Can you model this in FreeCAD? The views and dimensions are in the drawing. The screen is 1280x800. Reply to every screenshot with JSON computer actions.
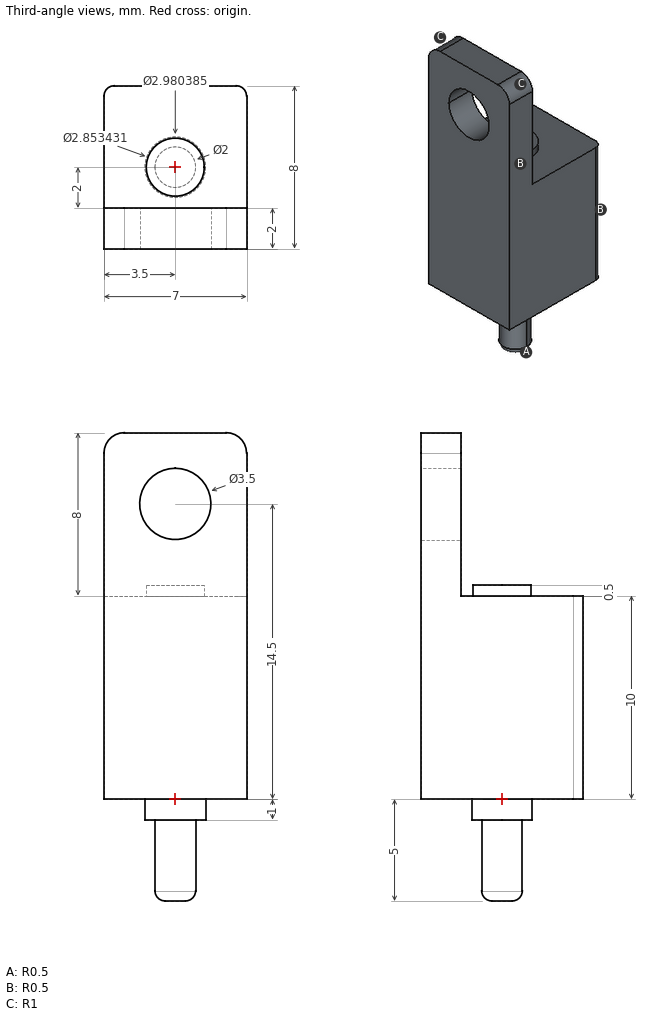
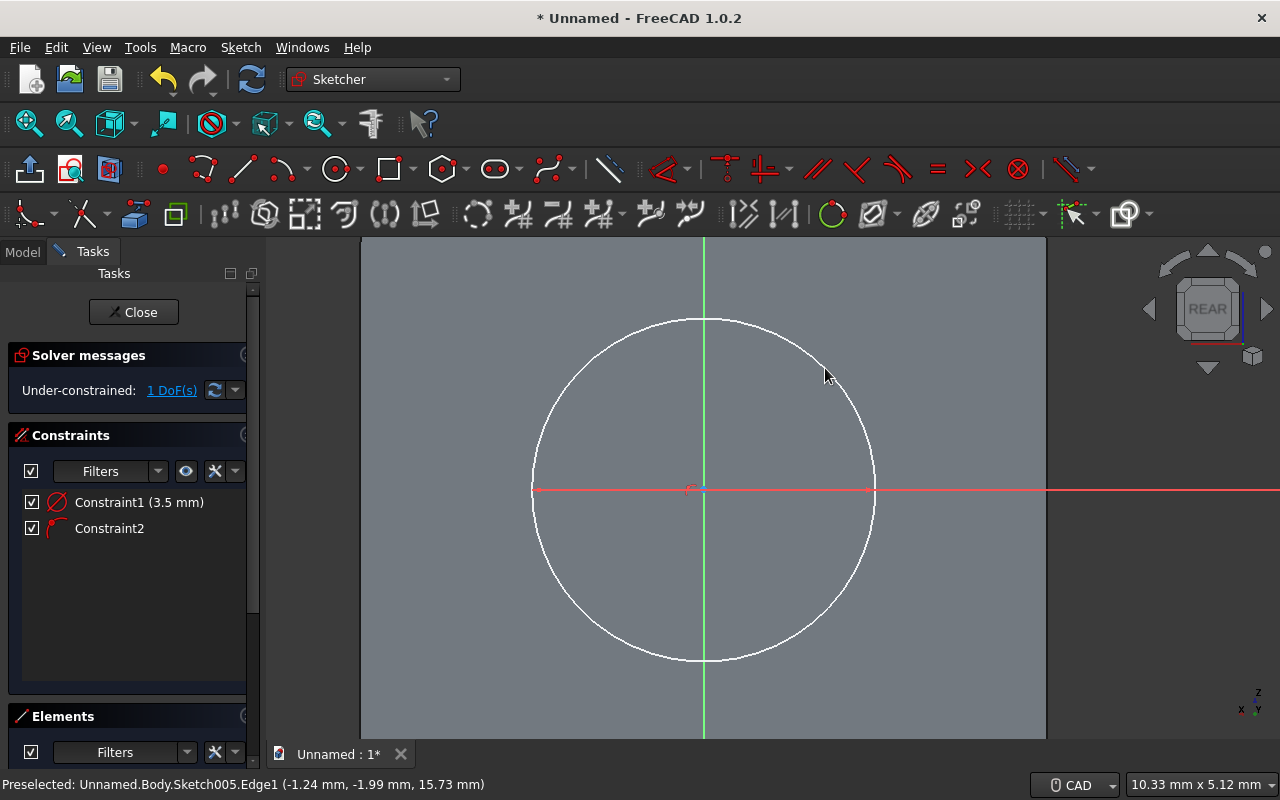
{"action": "key", "text": "d"}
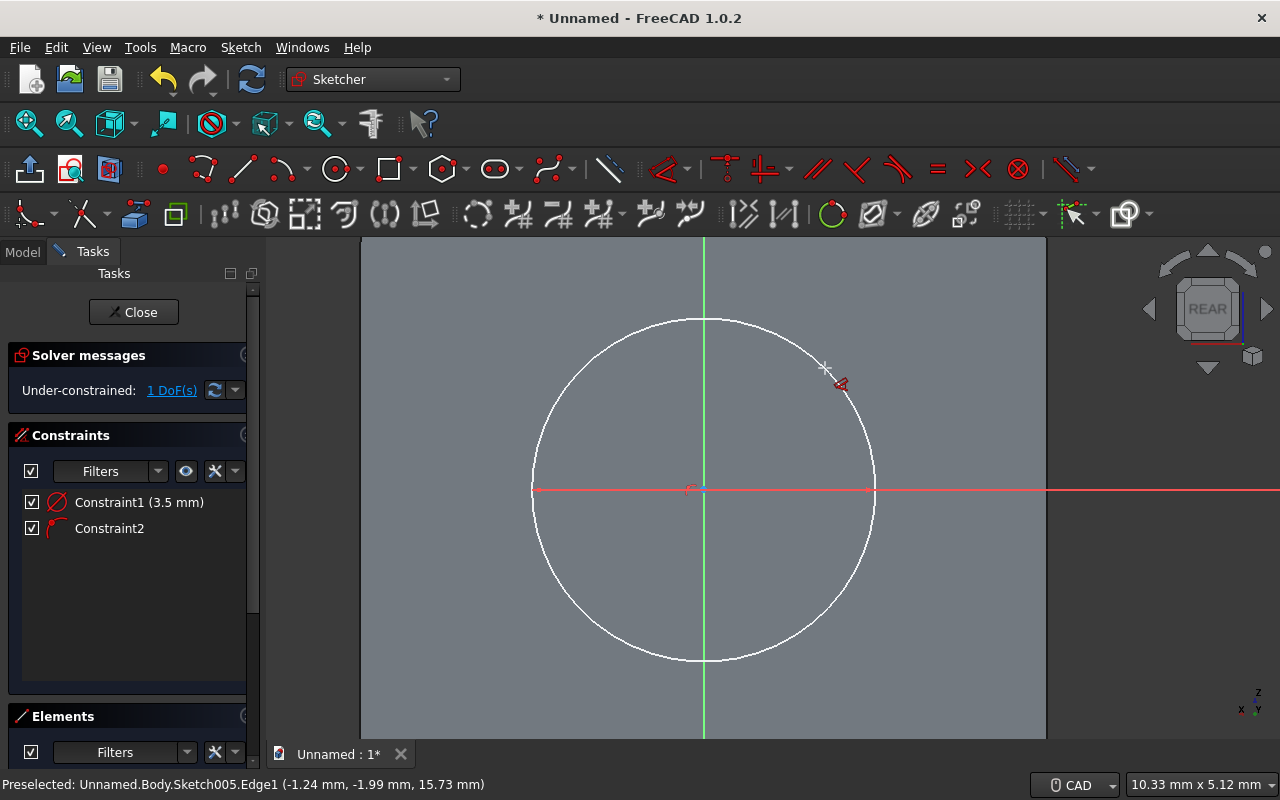
{"action": "left_click", "coordinate": [704, 490]}
{"action": "left_click", "coordinate": [738, 601]}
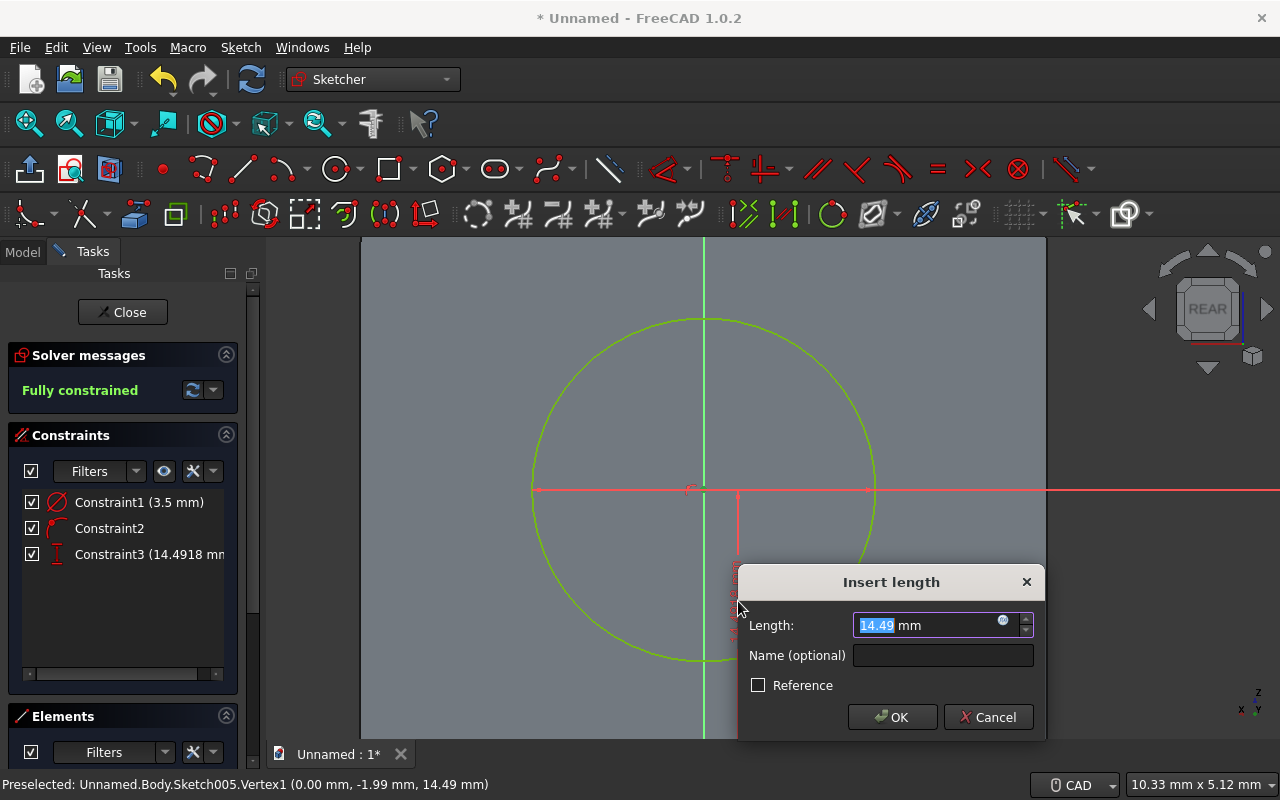
{"action": "type", "text": "14.5"}
{"action": "key", "text": "Return"}
{"action": "key", "text": "Escape"}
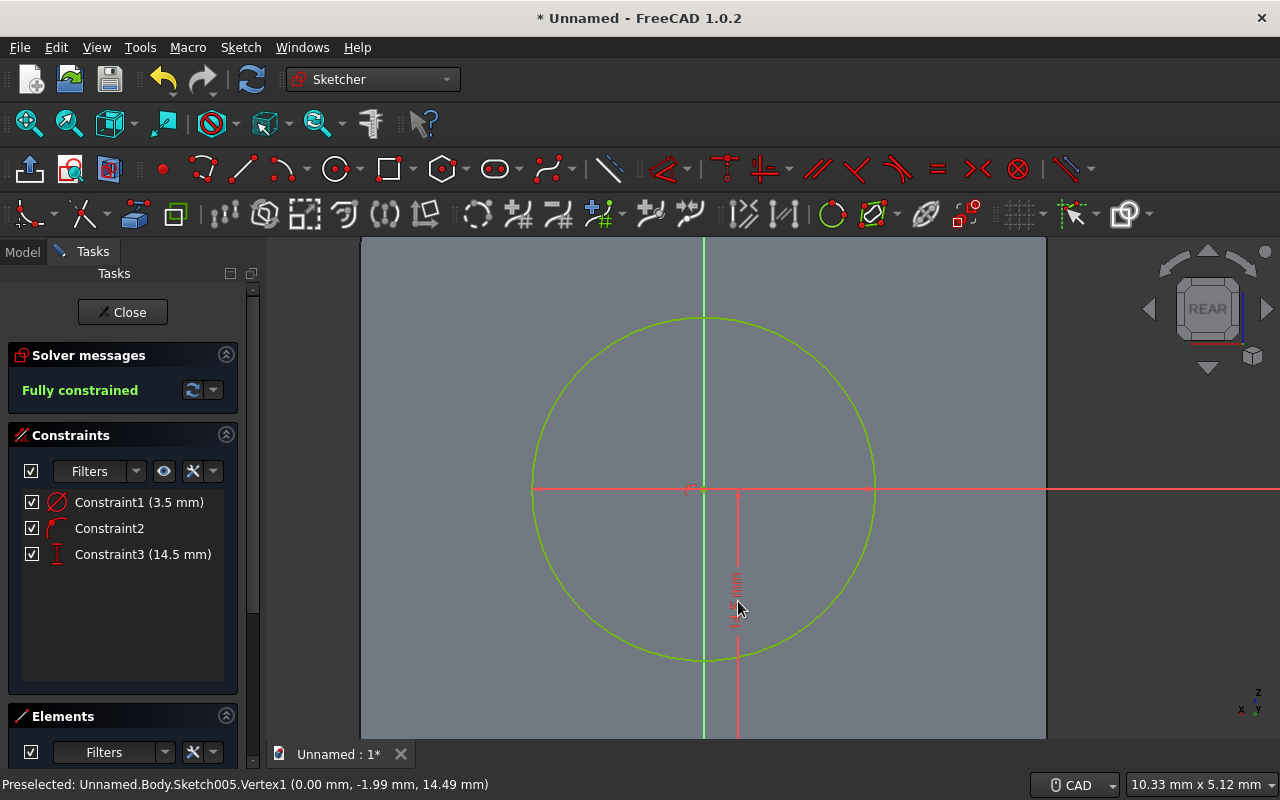
{"action": "left_click", "coordinate": [123, 312]}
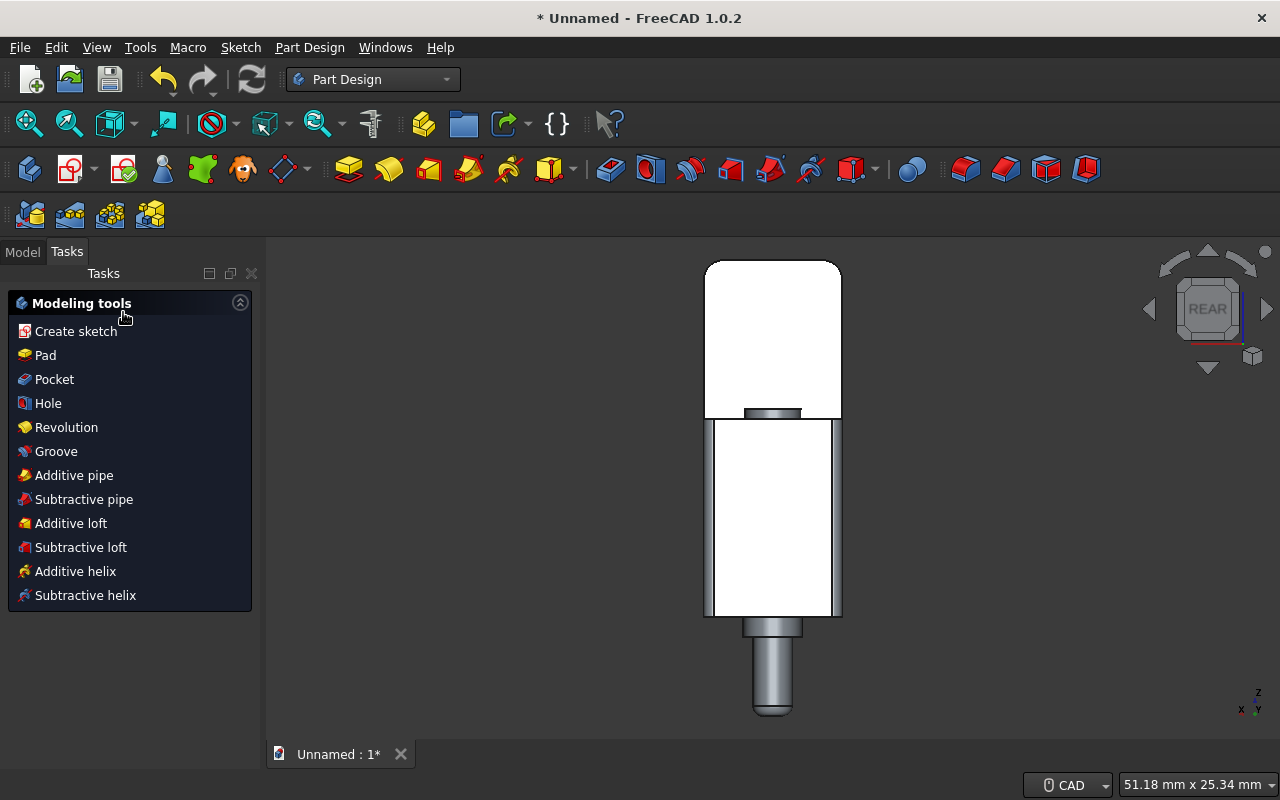
{"action": "left_click", "coordinate": [612, 170]}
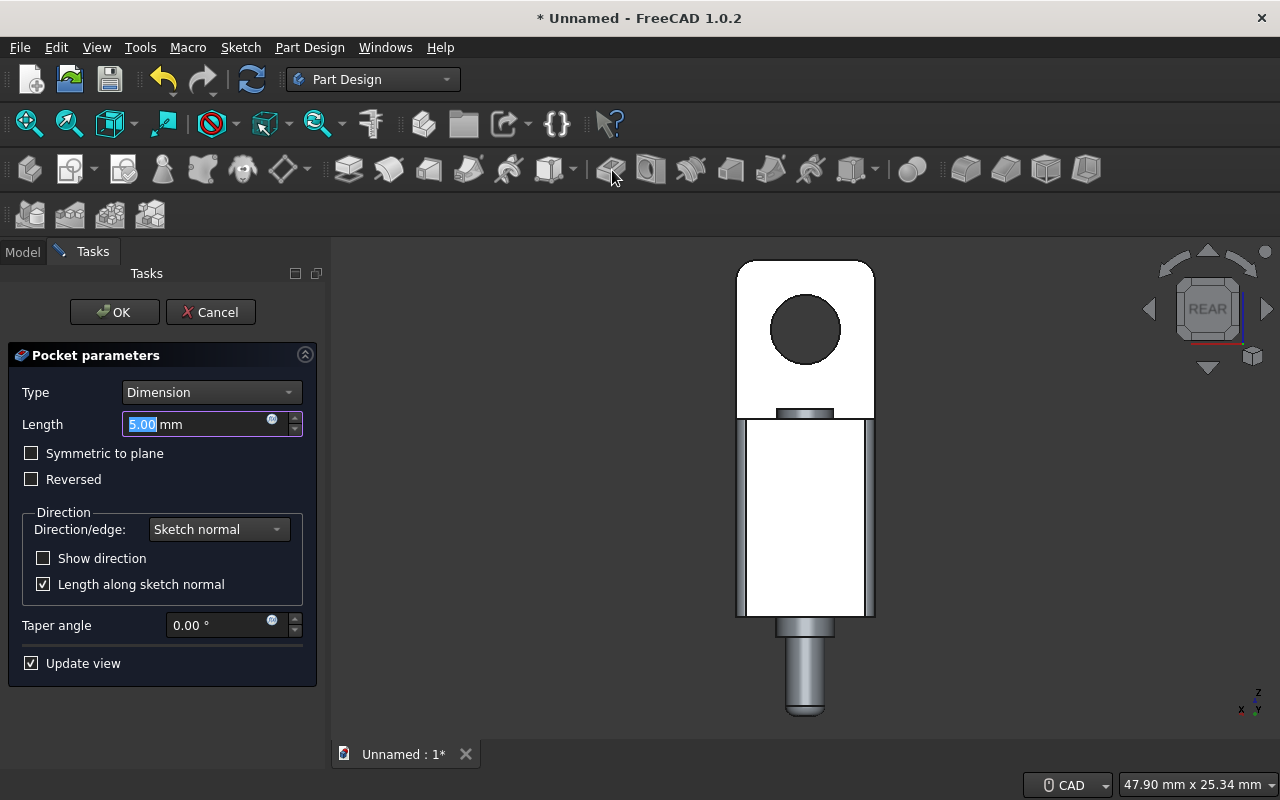
{"action": "left_click", "coordinate": [212, 392]}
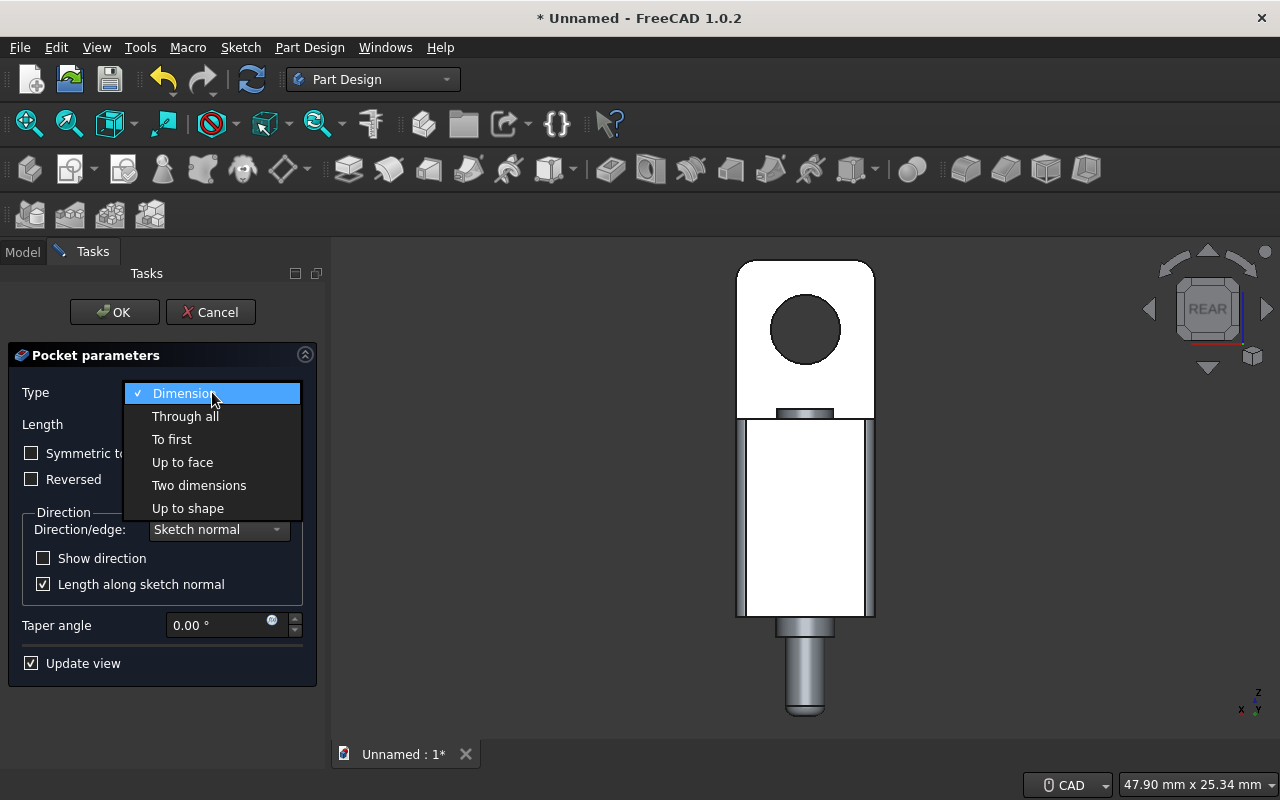
{"action": "left_click", "coordinate": [212, 416]}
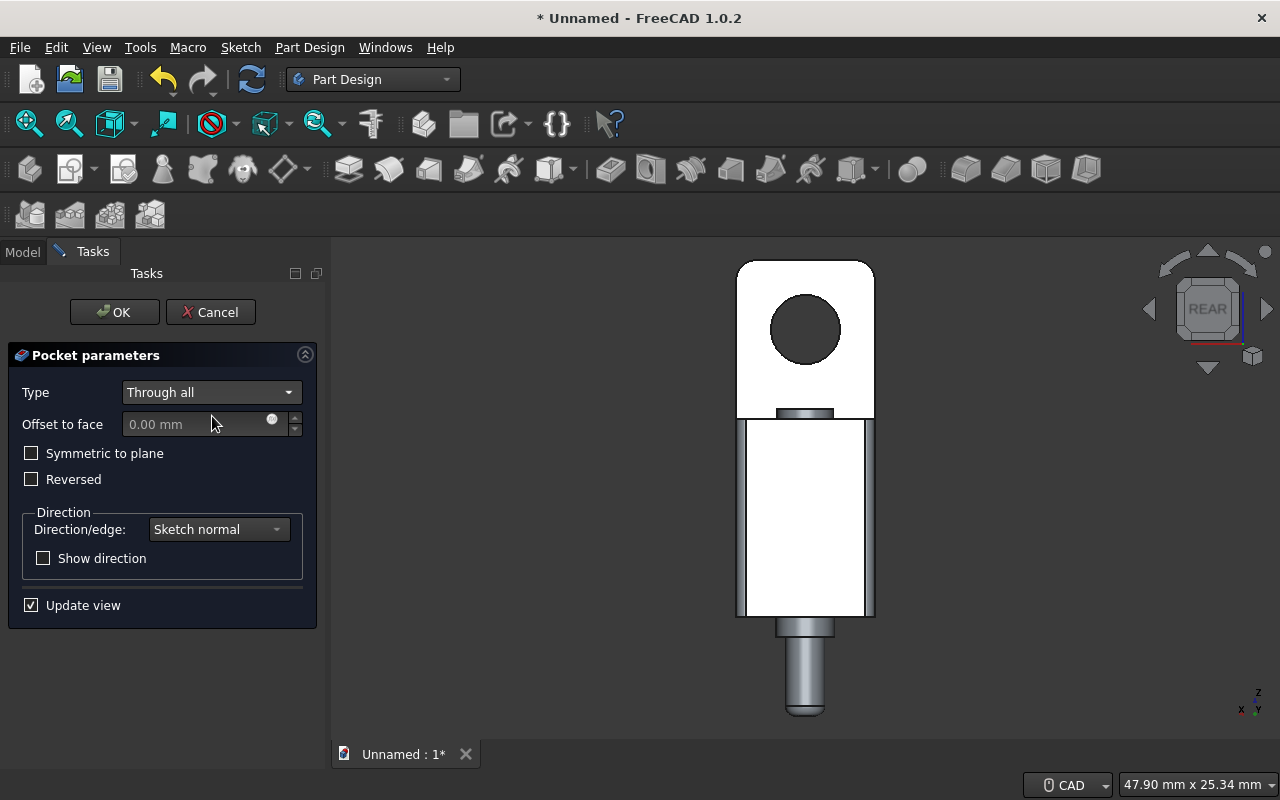
{"action": "left_click", "coordinate": [115, 312]}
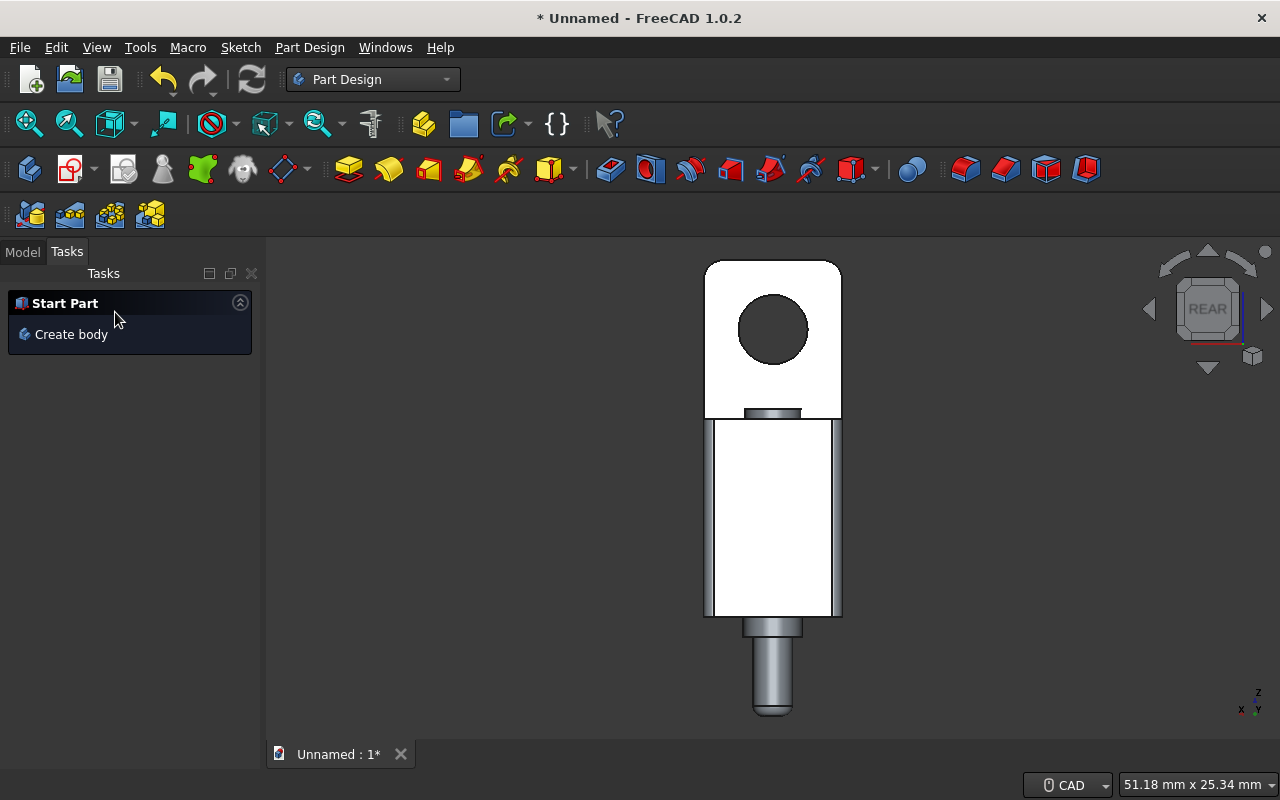
{"action": "key", "text": "0"}